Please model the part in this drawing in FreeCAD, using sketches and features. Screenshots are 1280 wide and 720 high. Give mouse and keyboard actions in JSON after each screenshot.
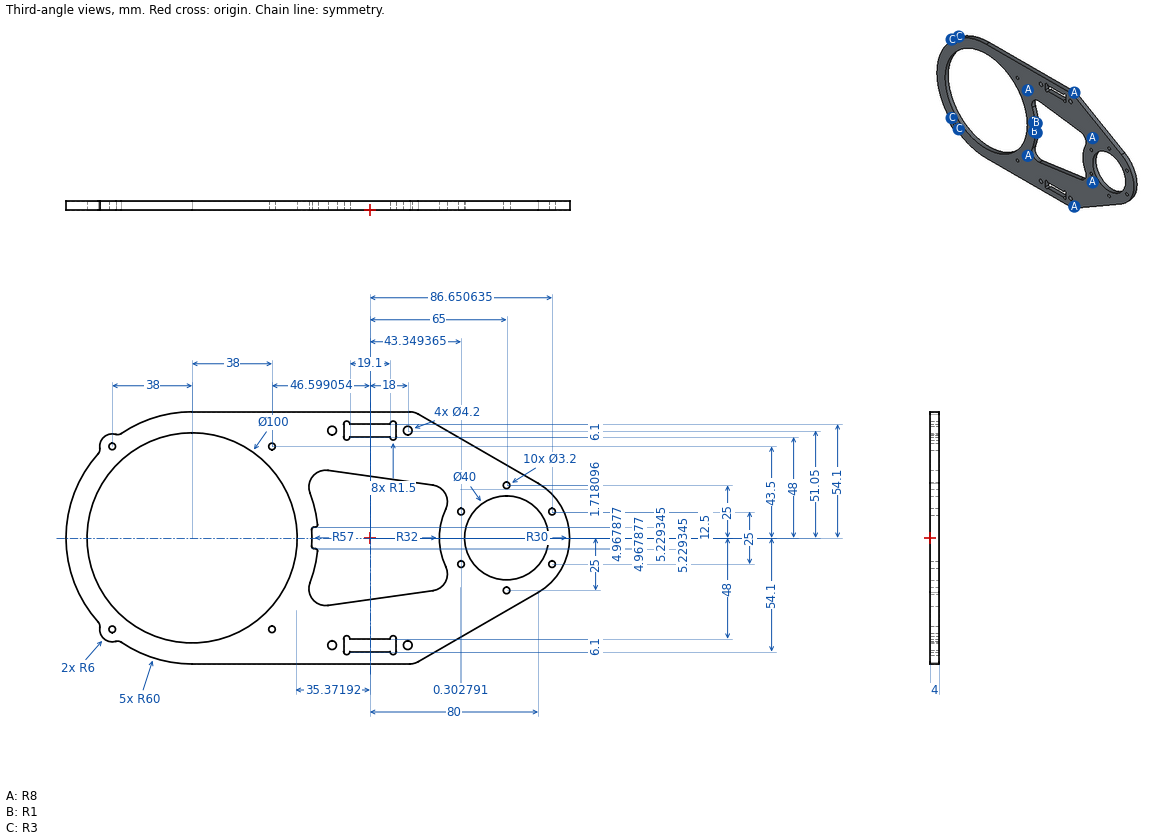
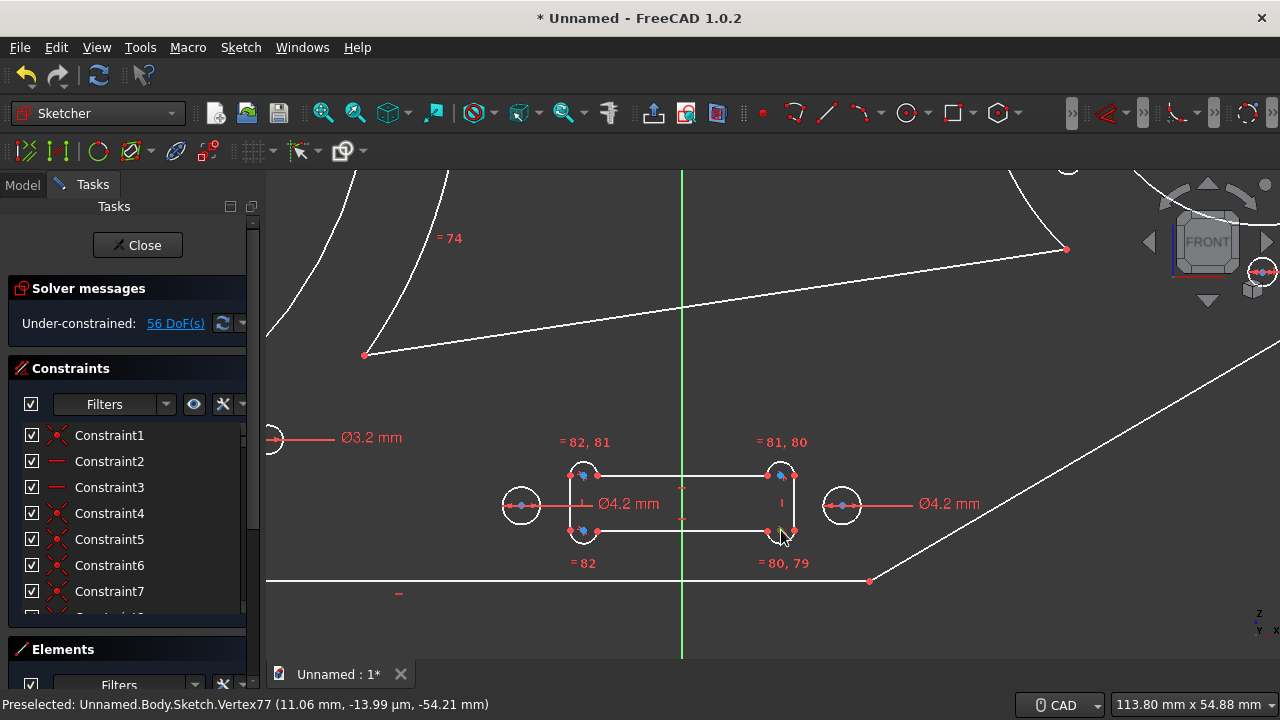
{"action": "scroll", "coordinate": [784, 535], "scroll_direction": "down", "scroll_amount": 7}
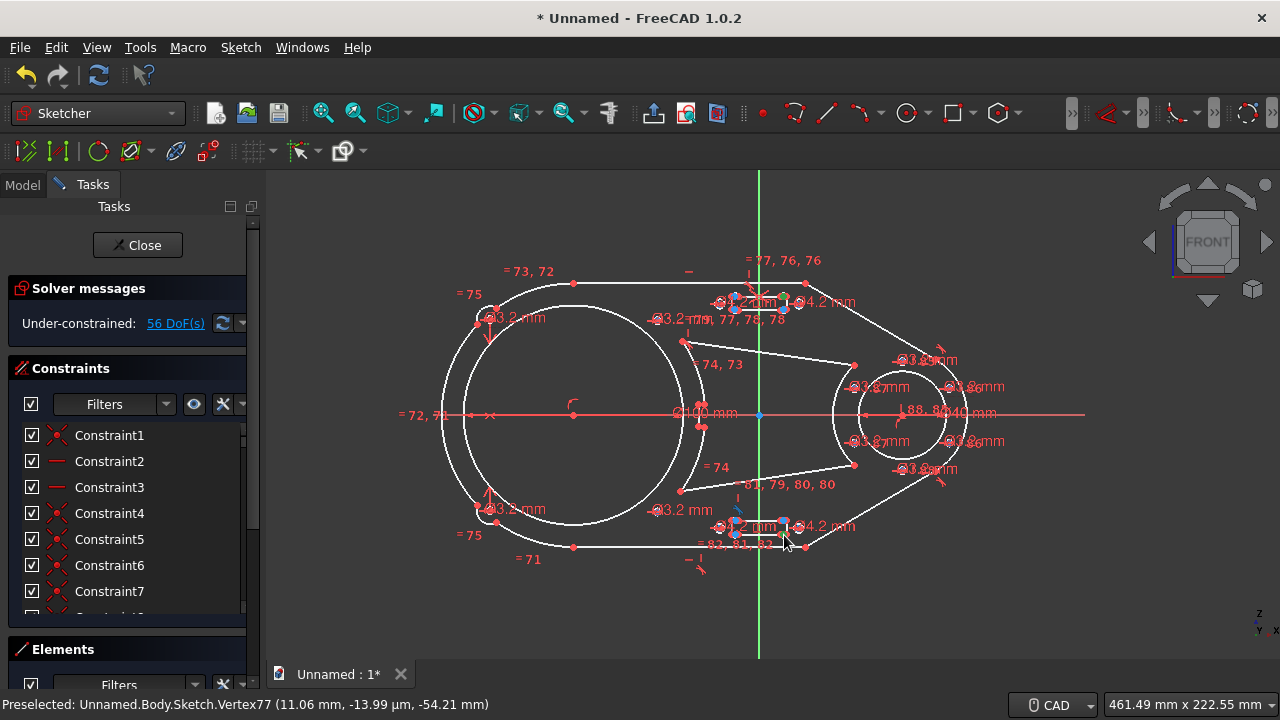
{"action": "left_click", "coordinate": [529, 415]}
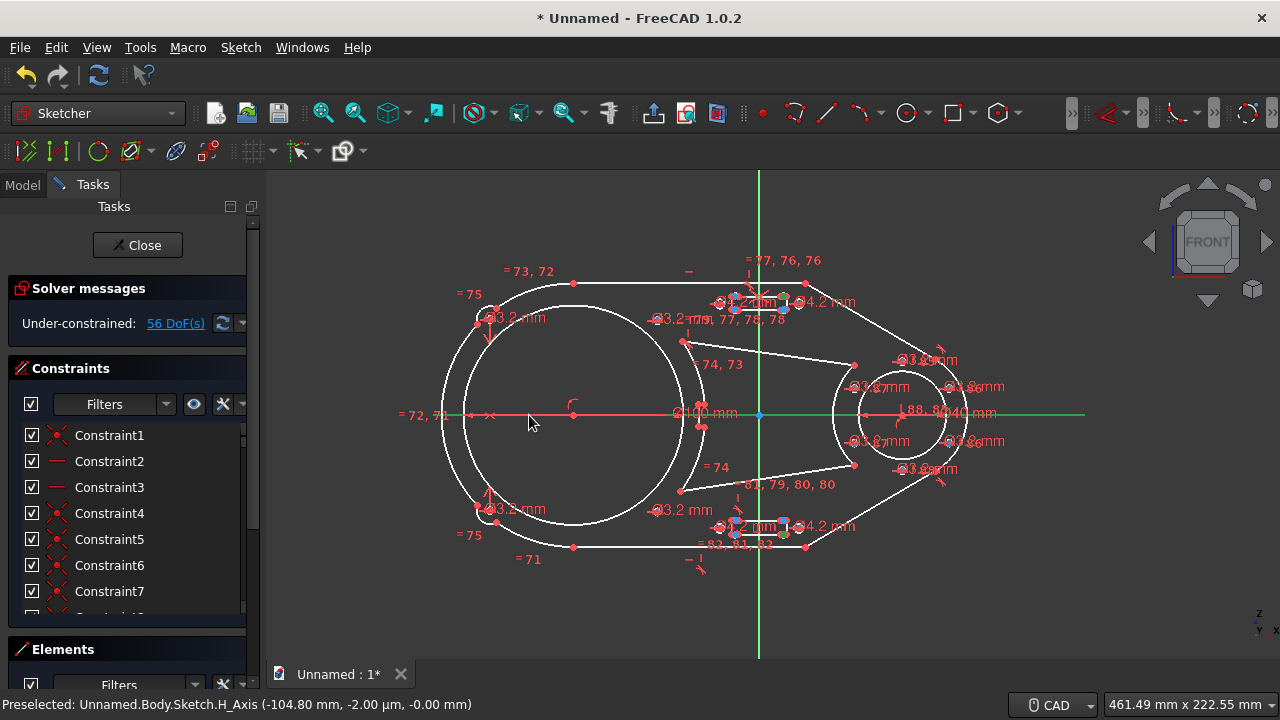
{"action": "key", "text": "s"}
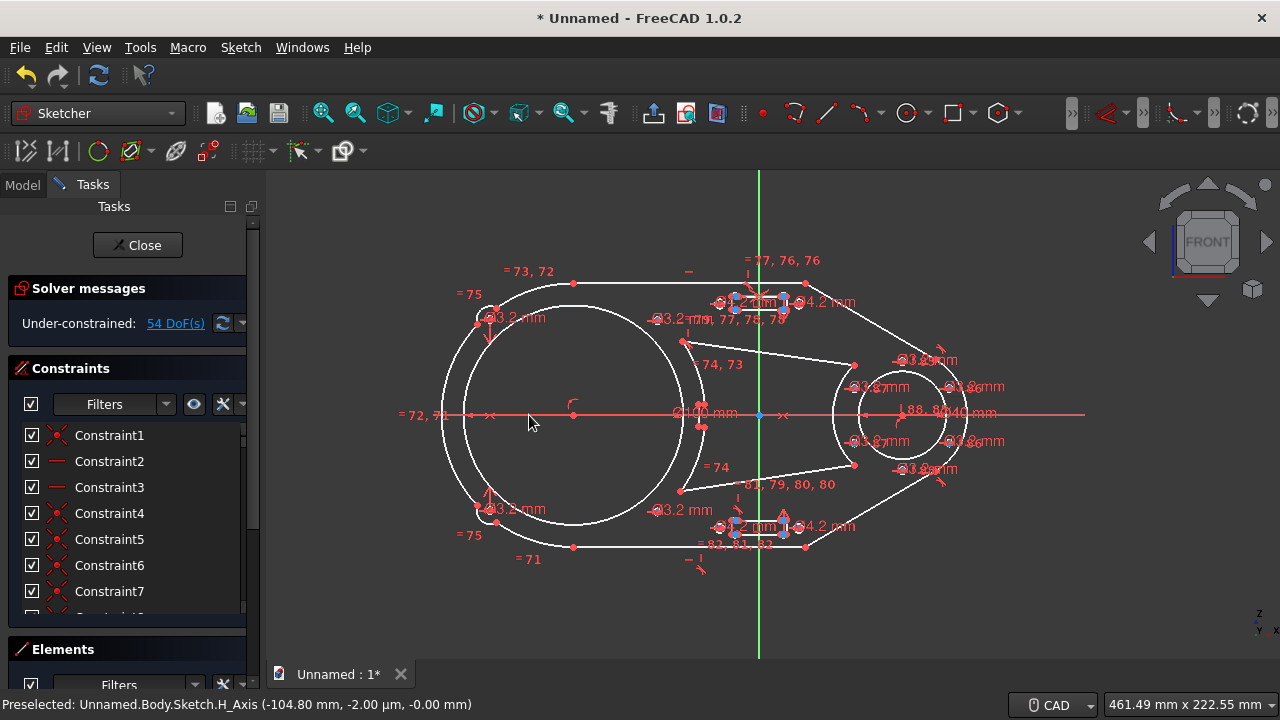
{"action": "scroll", "coordinate": [735, 310], "scroll_direction": "up", "scroll_amount": 7}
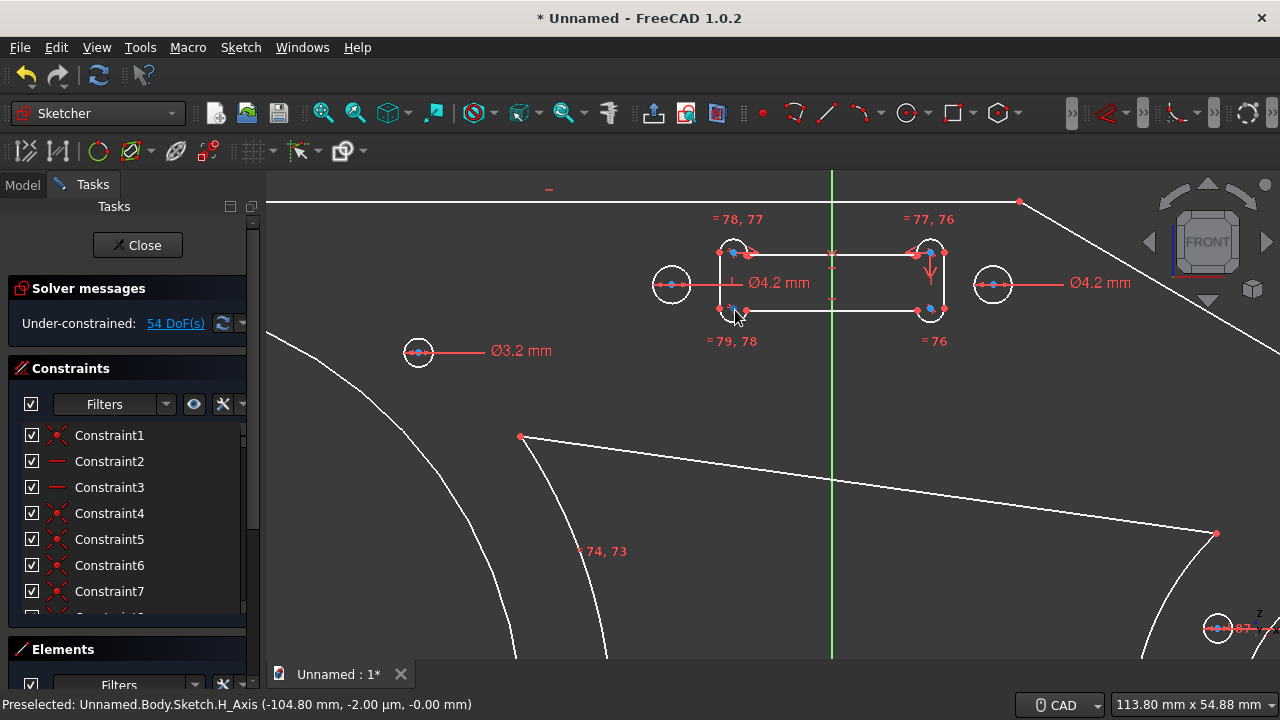
{"action": "left_click", "coordinate": [734, 309]}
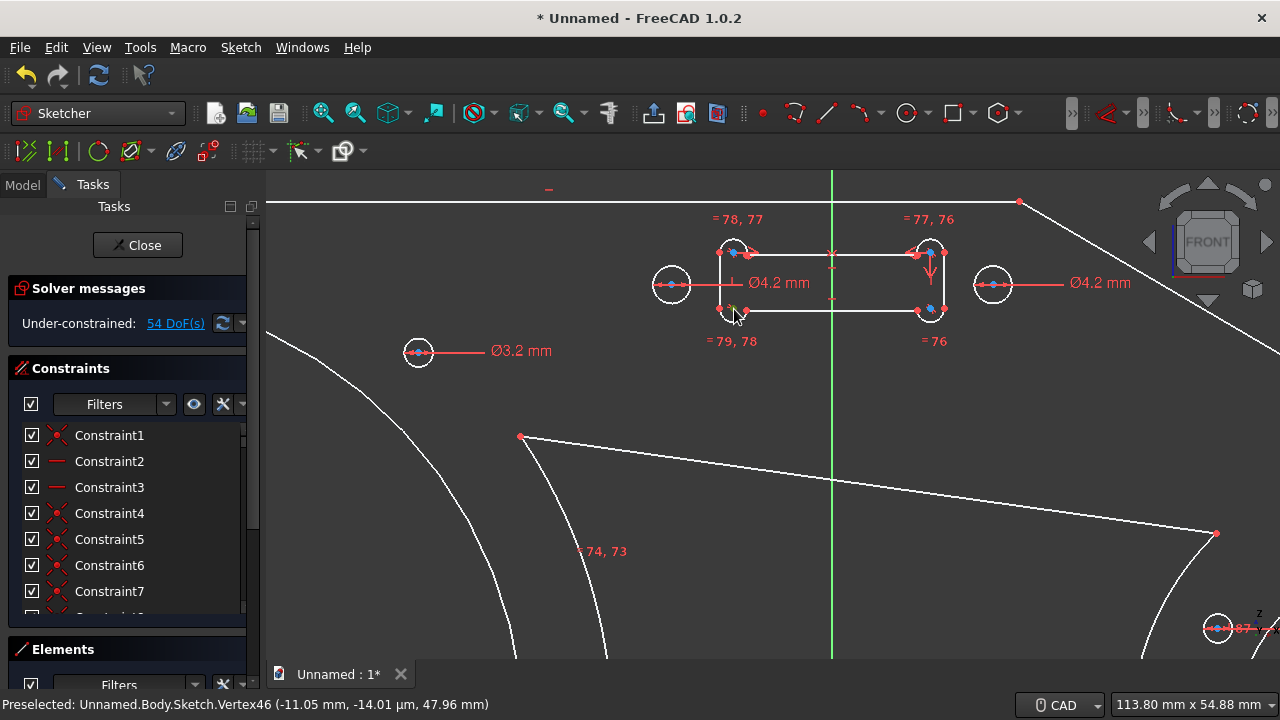
{"action": "scroll", "coordinate": [735, 309], "scroll_direction": "down", "scroll_amount": 7}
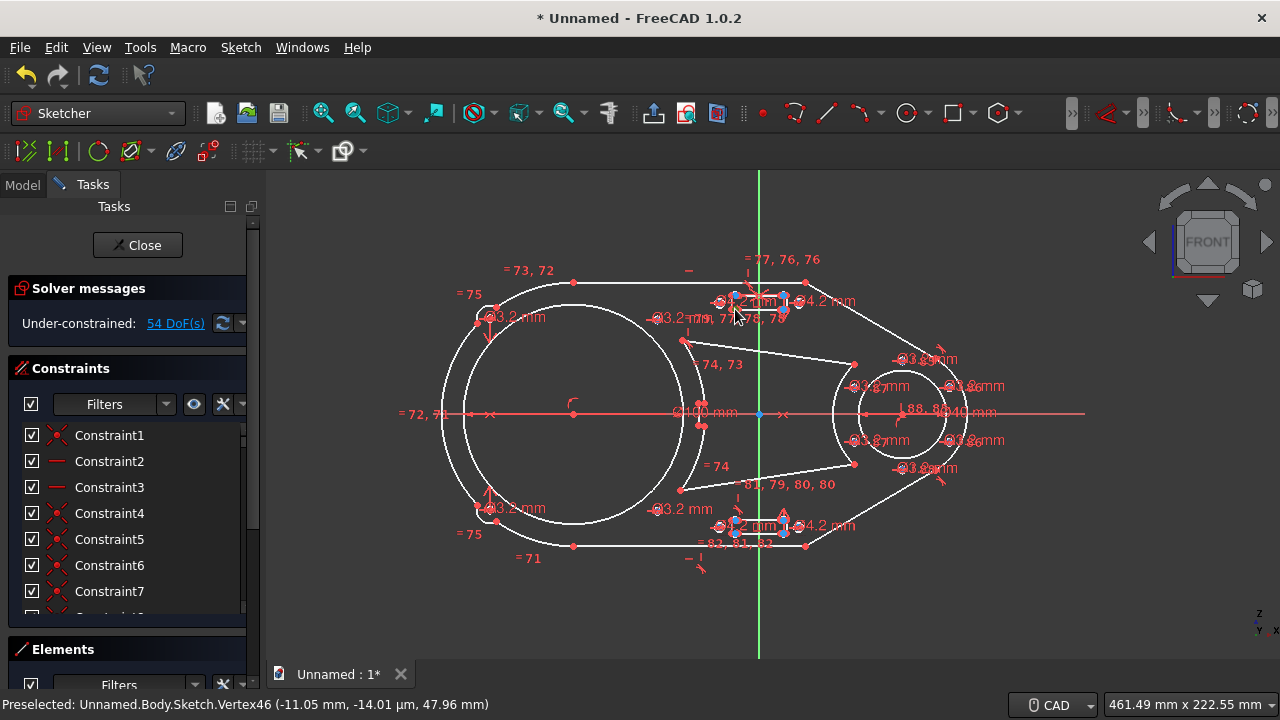
{"action": "scroll", "coordinate": [735, 520], "scroll_direction": "up", "scroll_amount": 7}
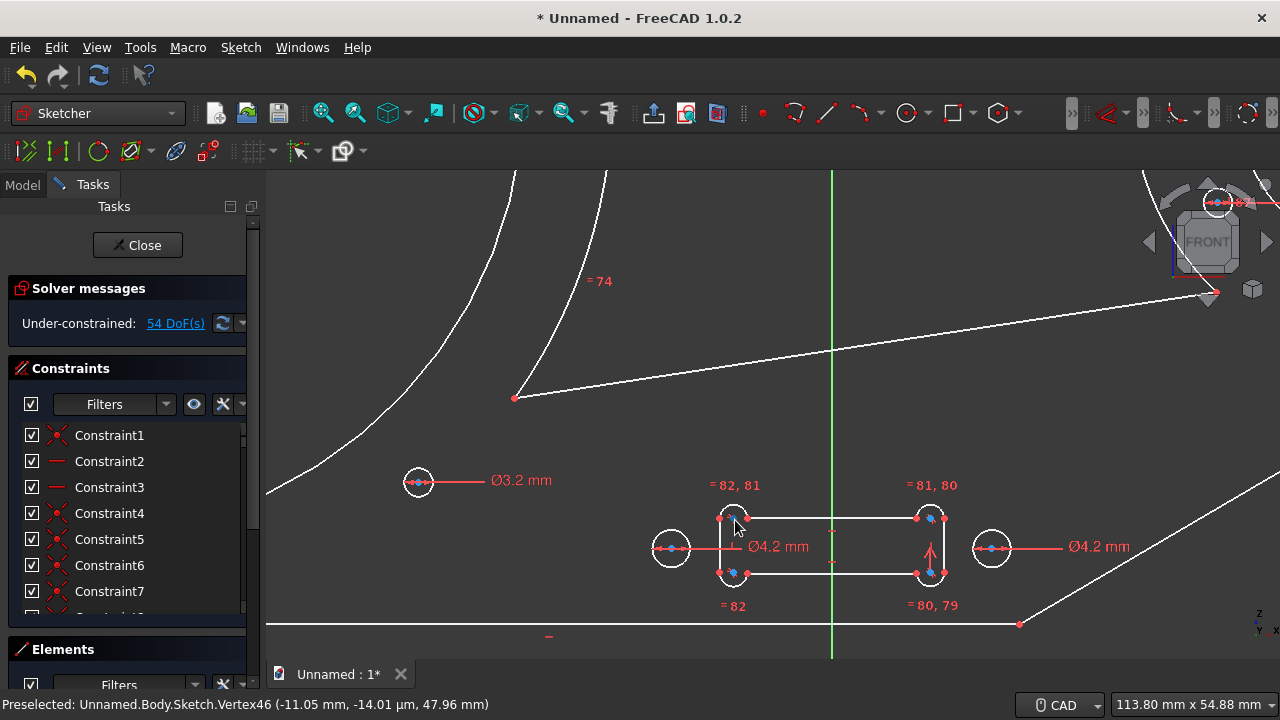
{"action": "left_click", "coordinate": [734, 518]}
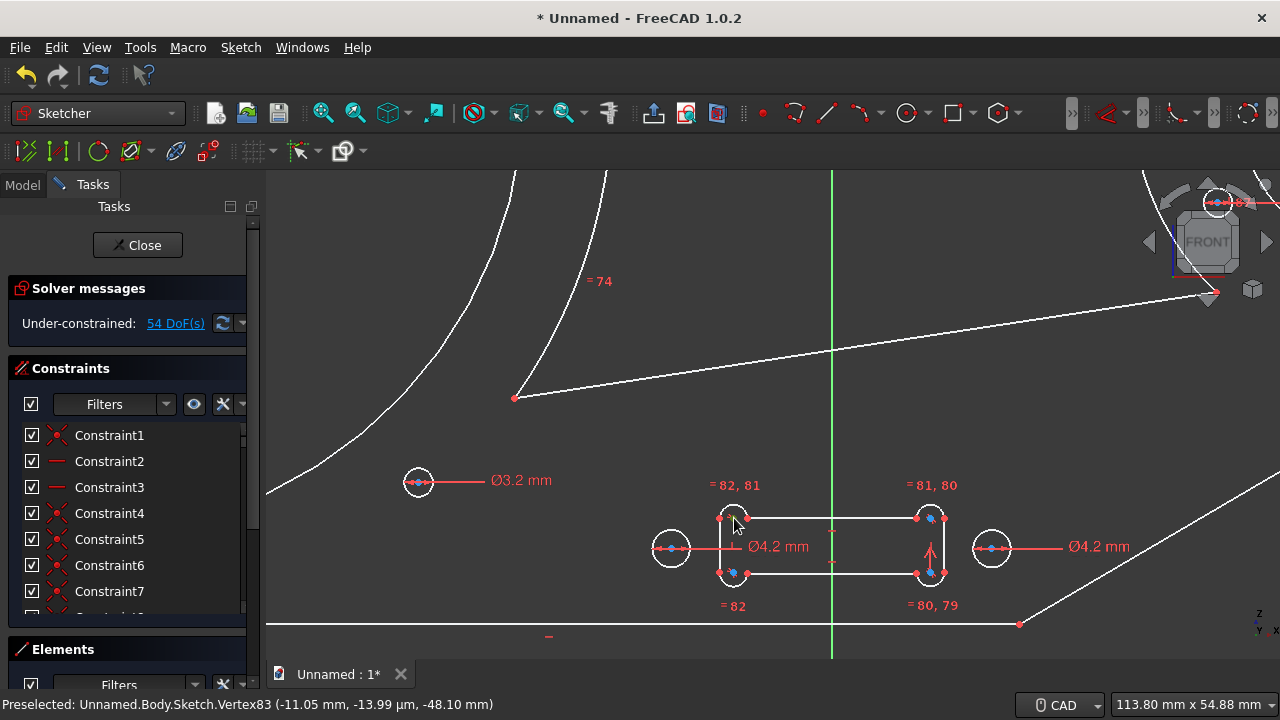
{"action": "scroll", "coordinate": [735, 521], "scroll_direction": "down", "scroll_amount": 7}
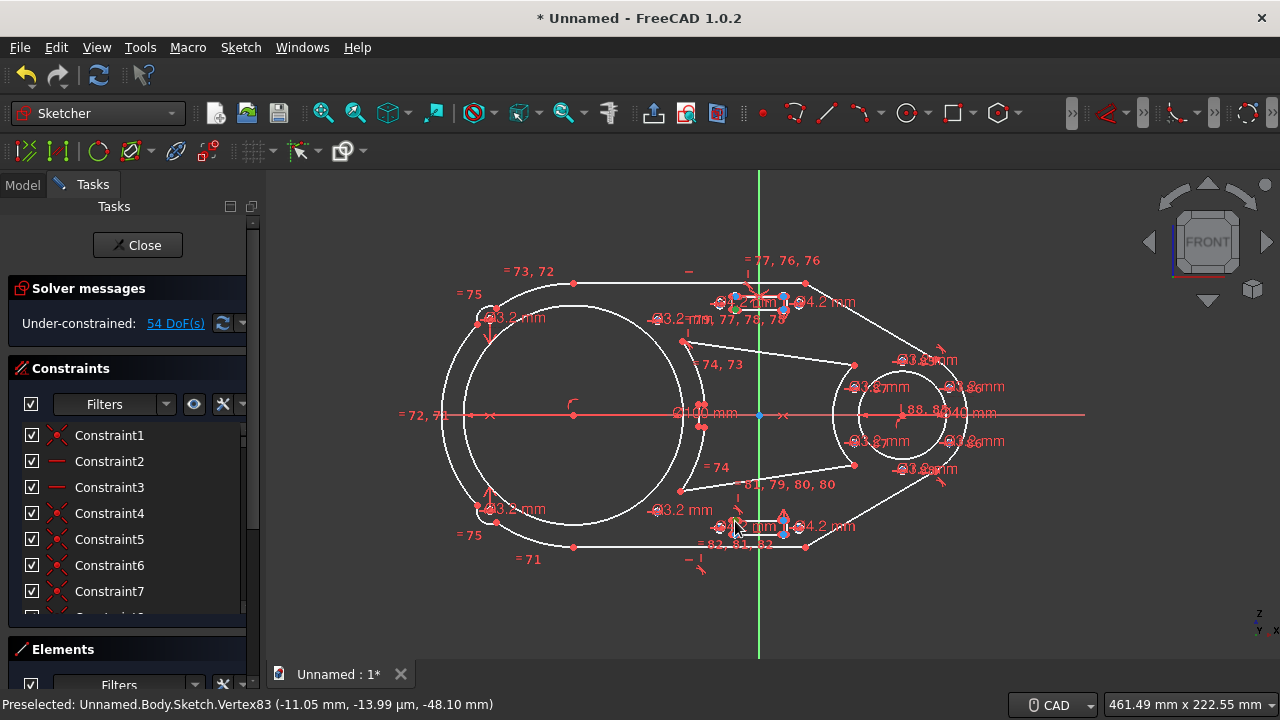
{"action": "left_click", "coordinate": [529, 415]}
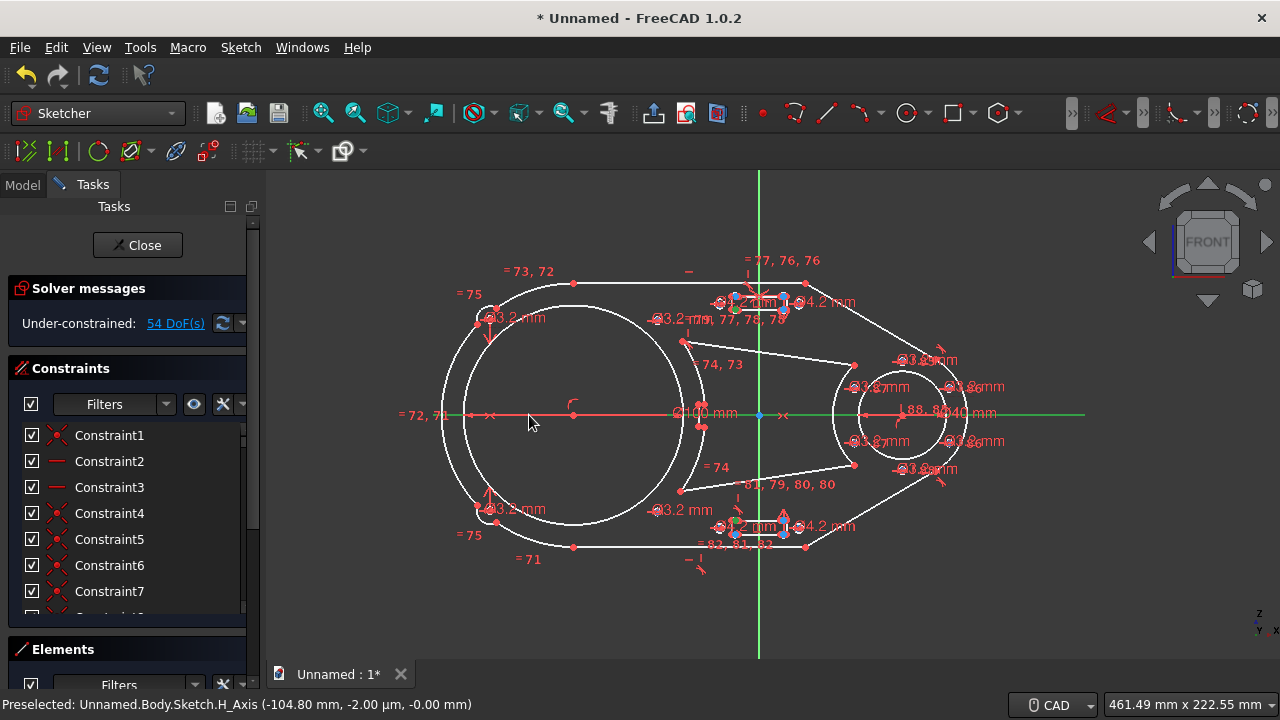
{"action": "key", "text": "s"}